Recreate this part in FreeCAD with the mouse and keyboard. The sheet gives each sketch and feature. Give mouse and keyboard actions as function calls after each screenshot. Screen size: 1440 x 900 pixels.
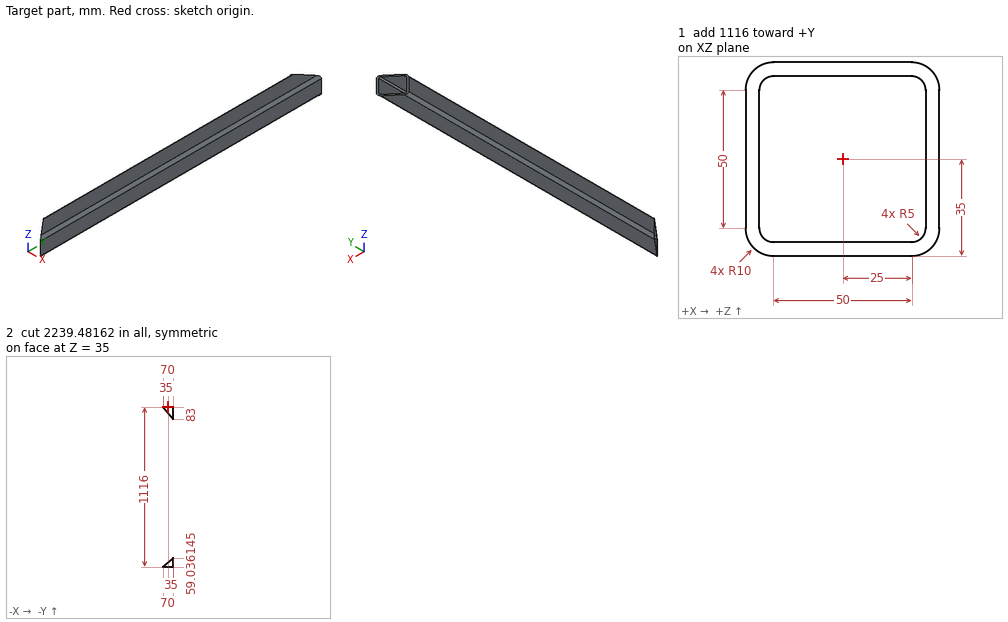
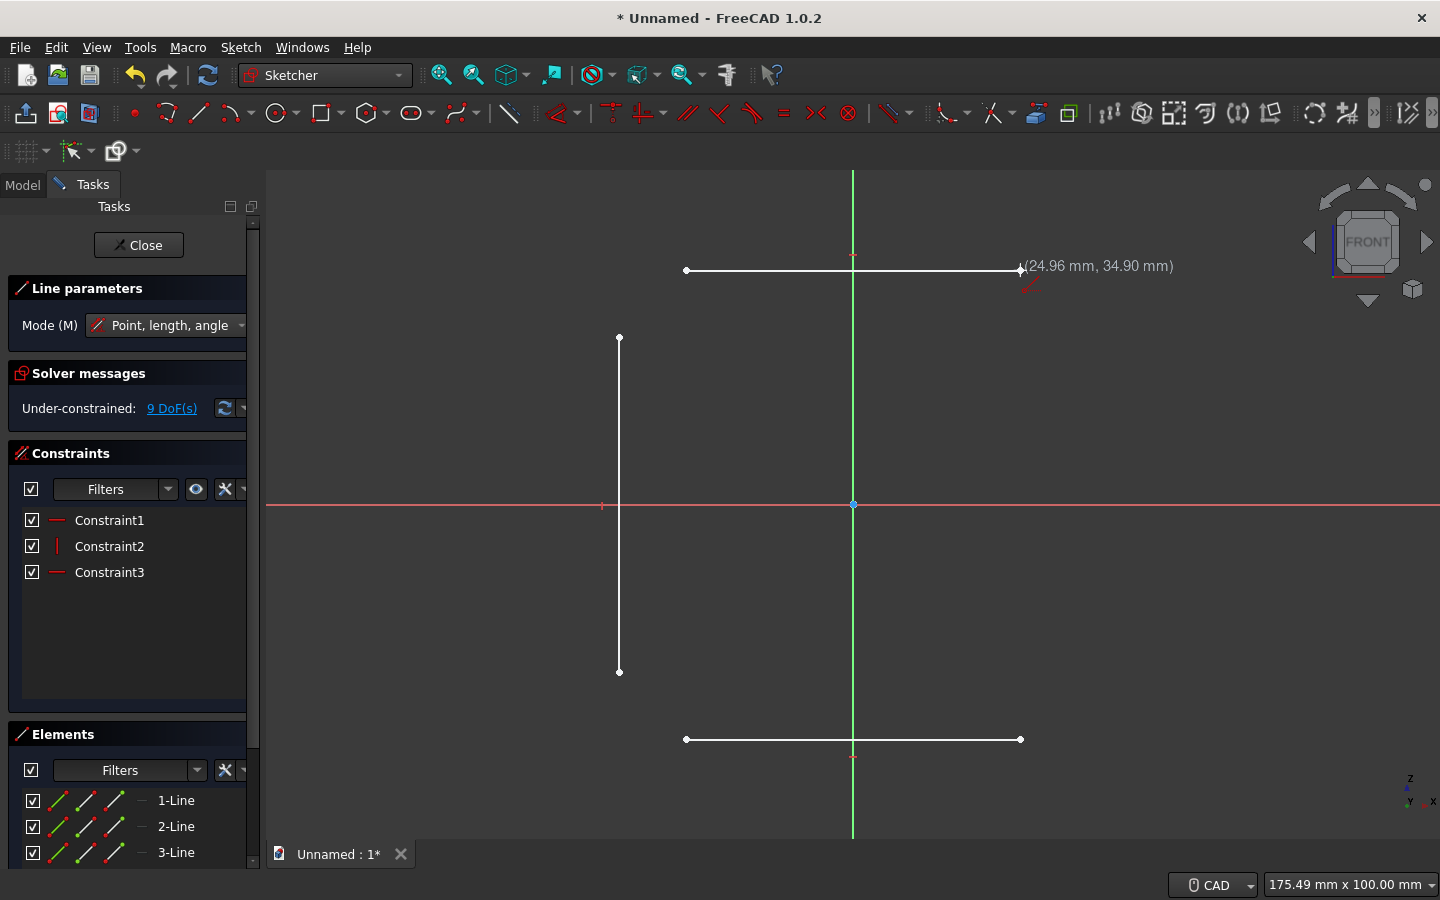
click(1087, 337)
click(1087, 672)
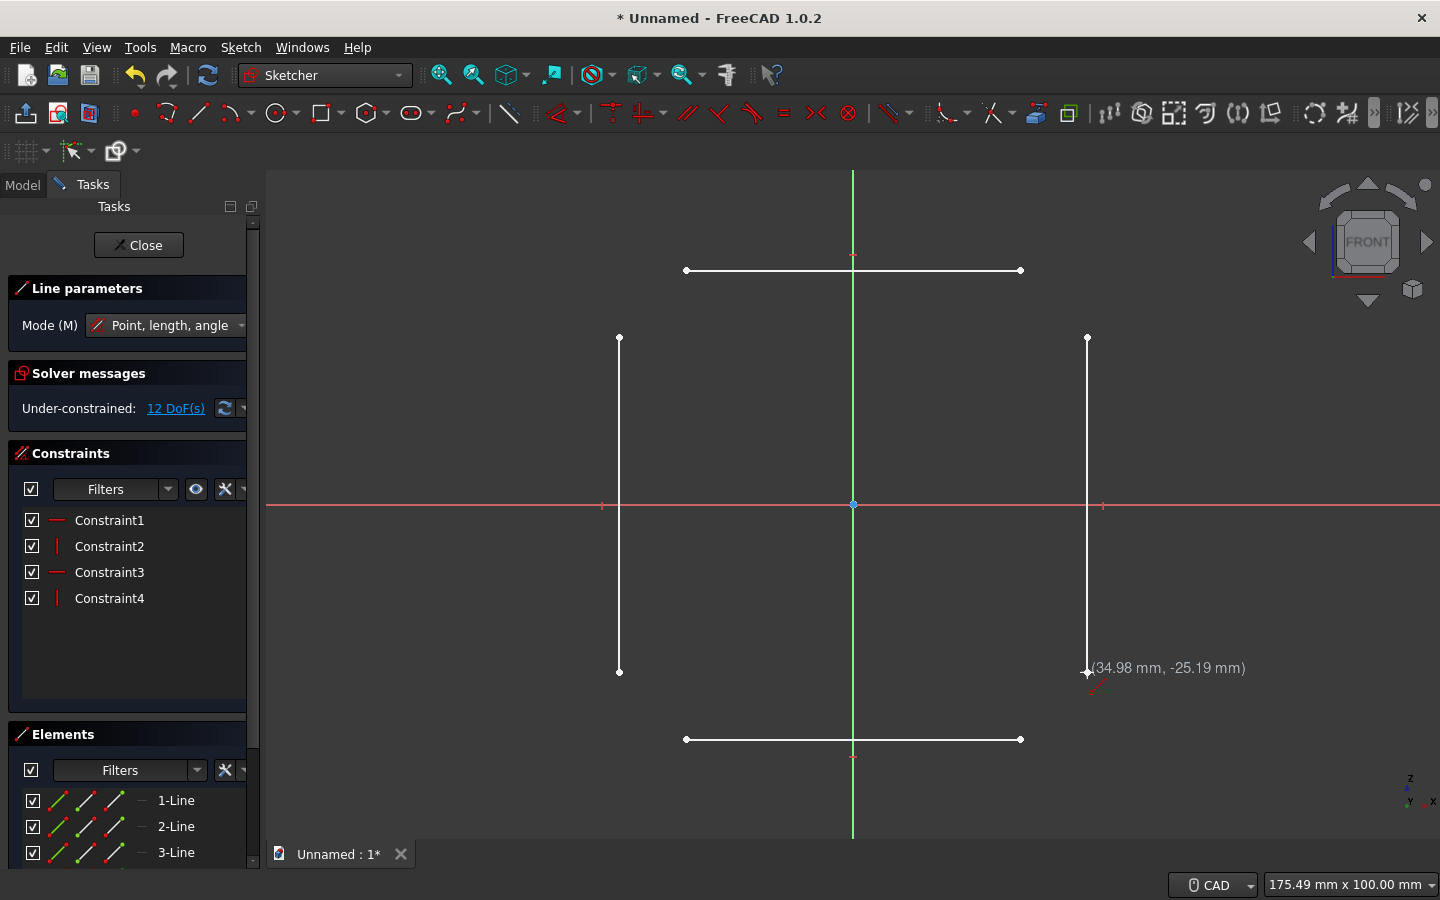
key(g)
key(3)
key(a)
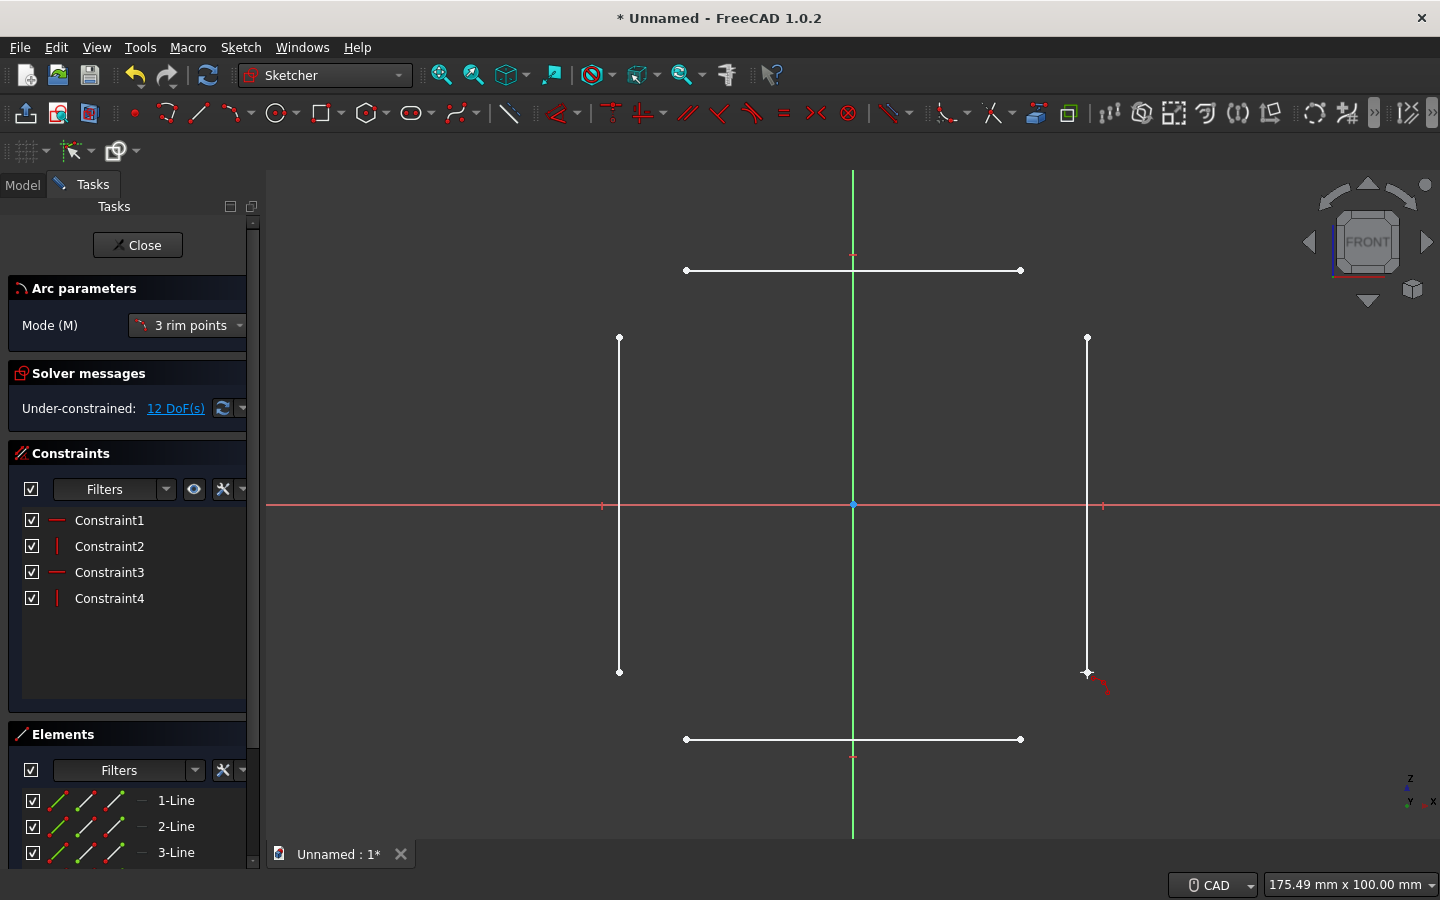
click(686, 740)
click(619, 673)
click(638, 719)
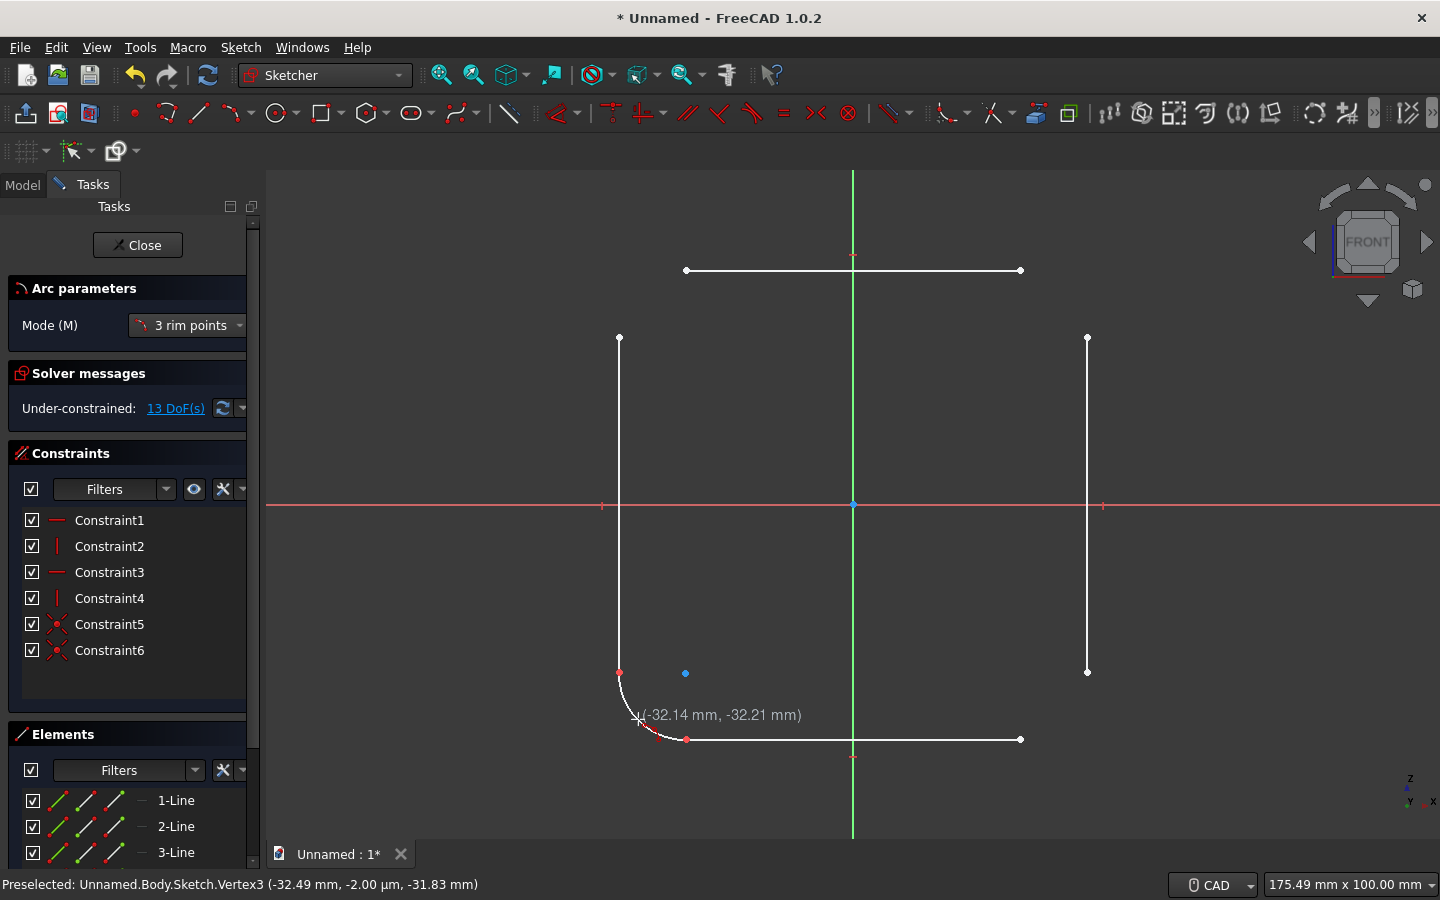
click(619, 338)
click(686, 271)
click(638, 290)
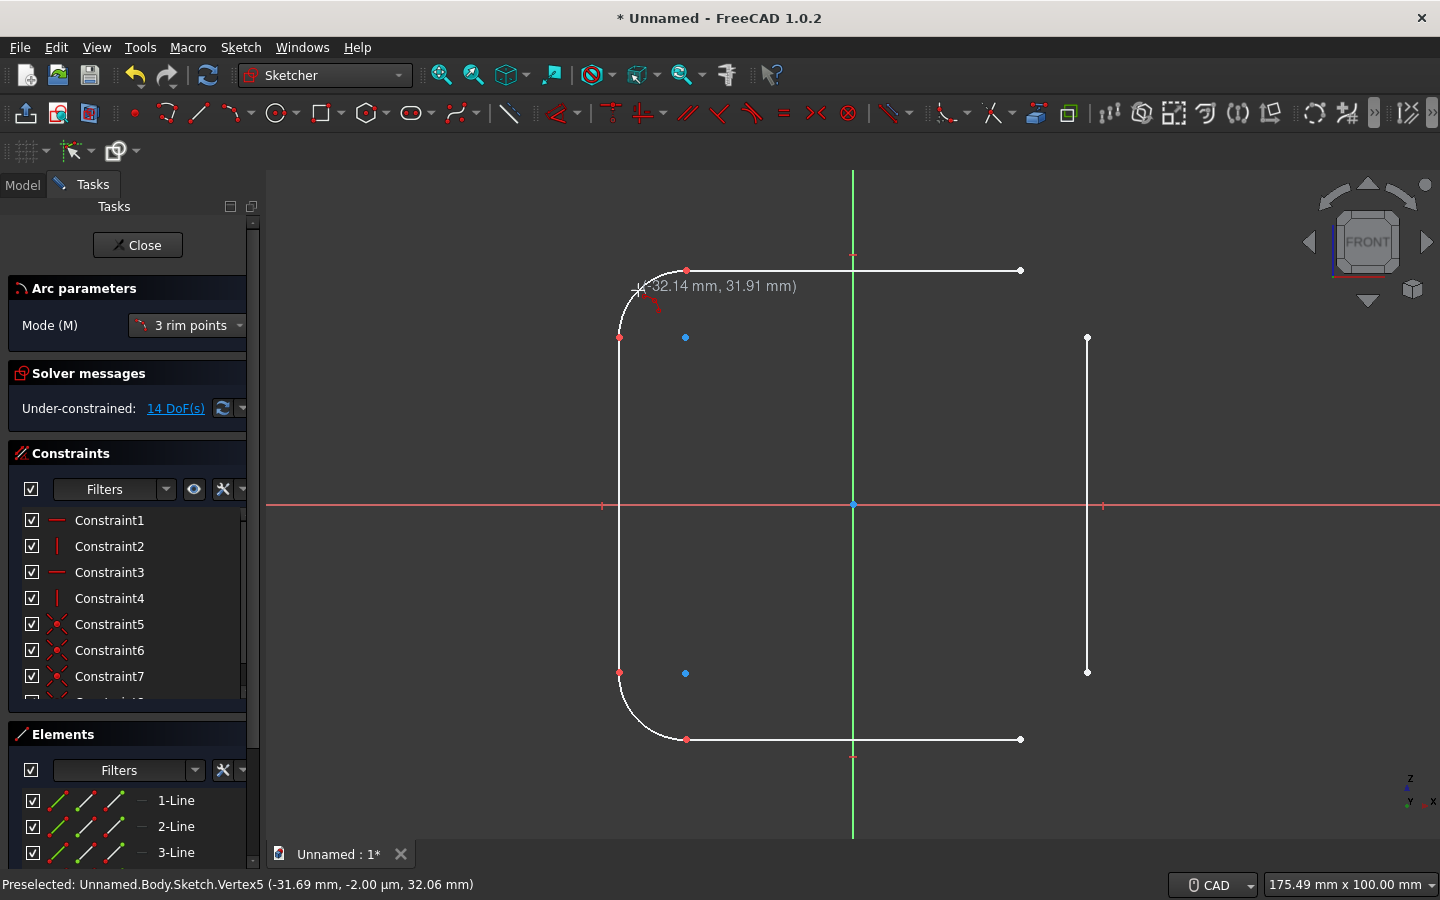
click(1020, 271)
click(1087, 338)
click(1068, 290)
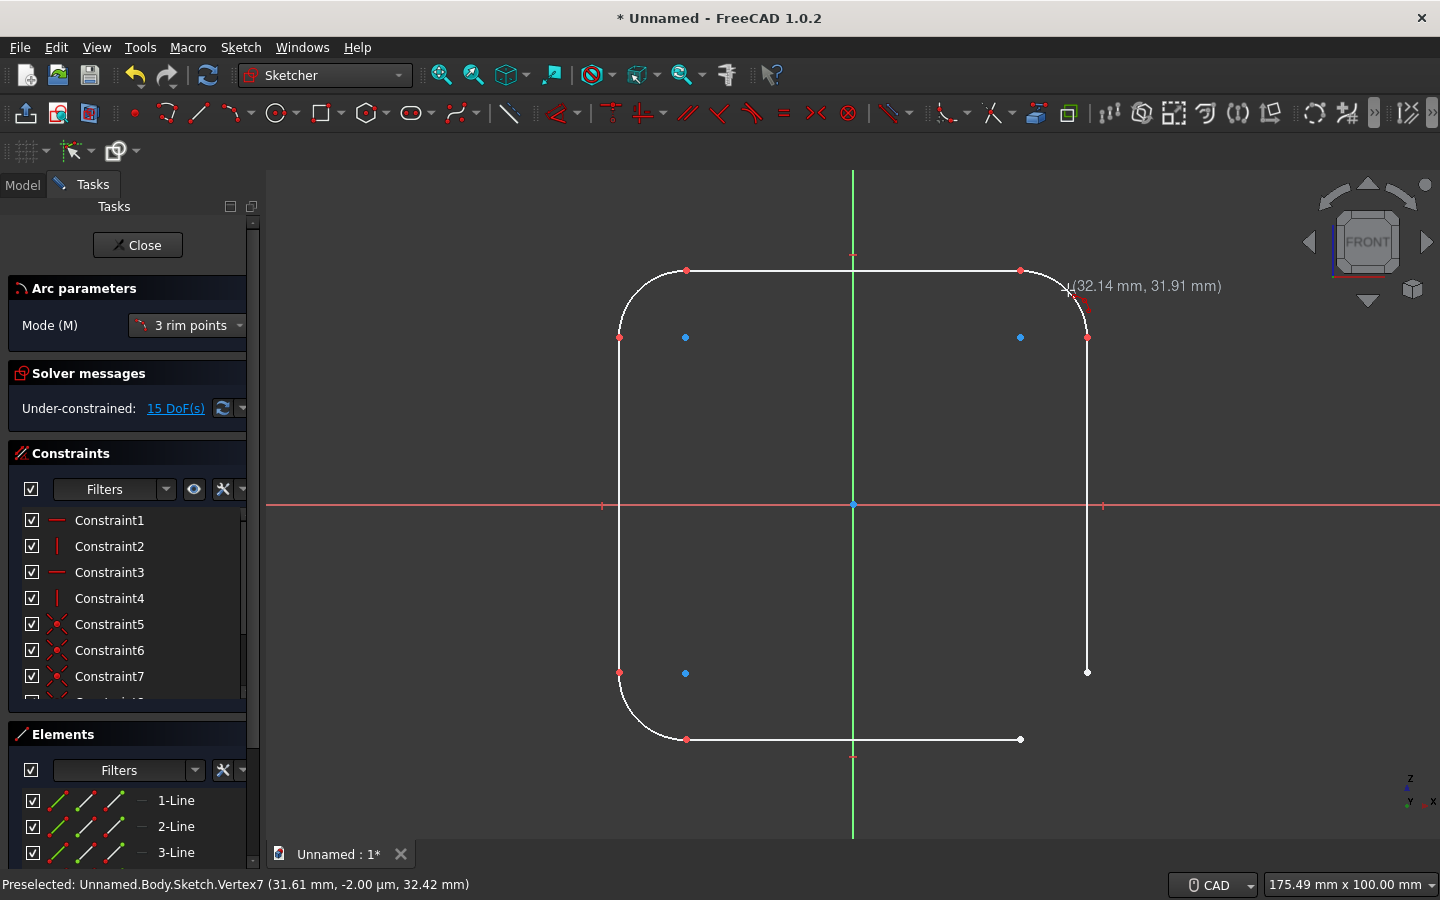
click(1087, 673)
click(1020, 740)
click(1068, 719)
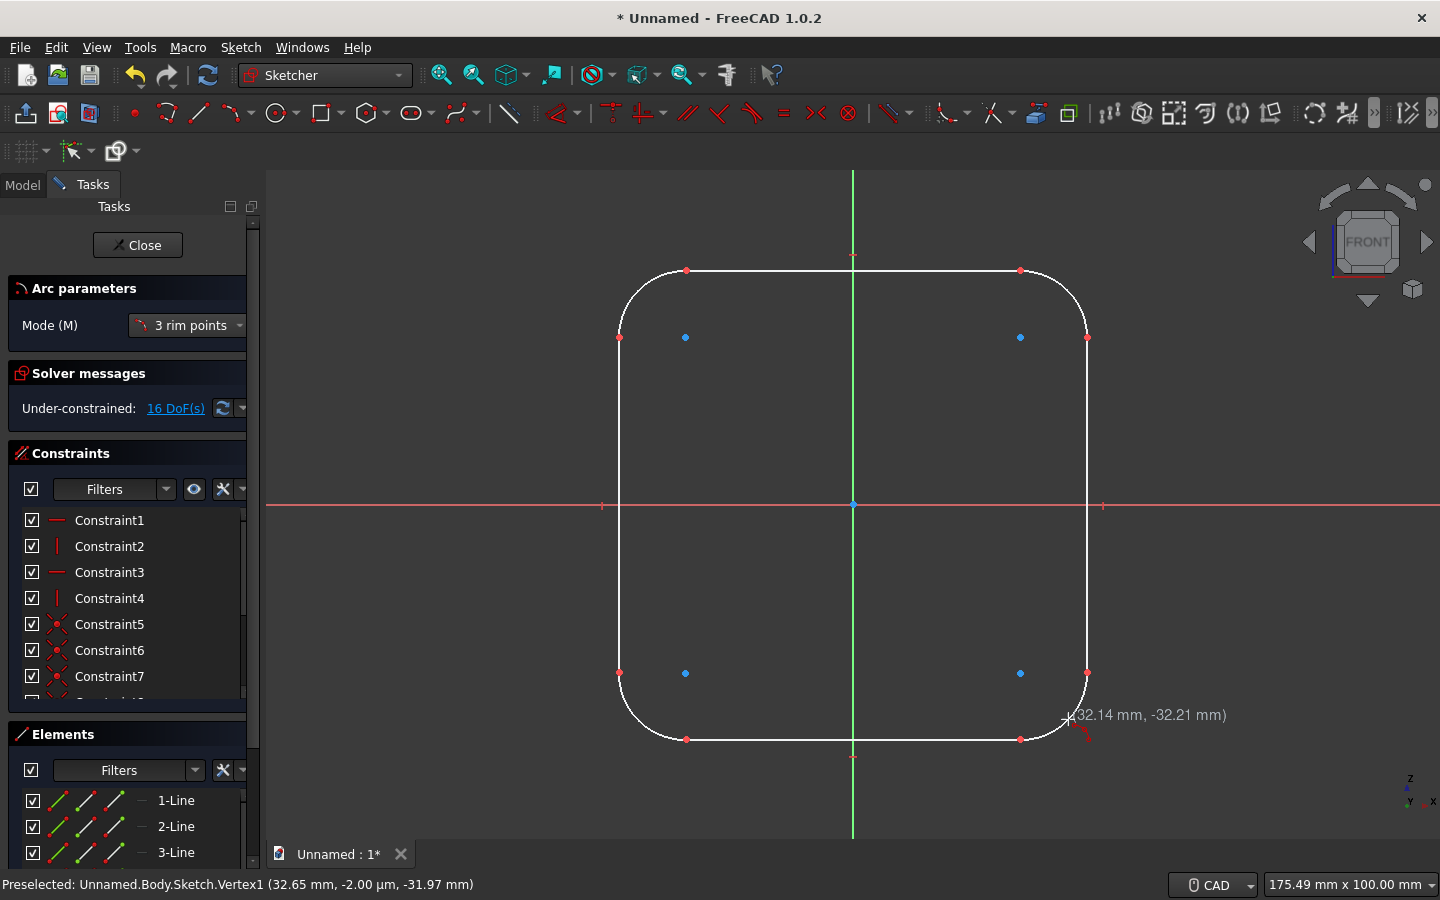
key(g)
key(l)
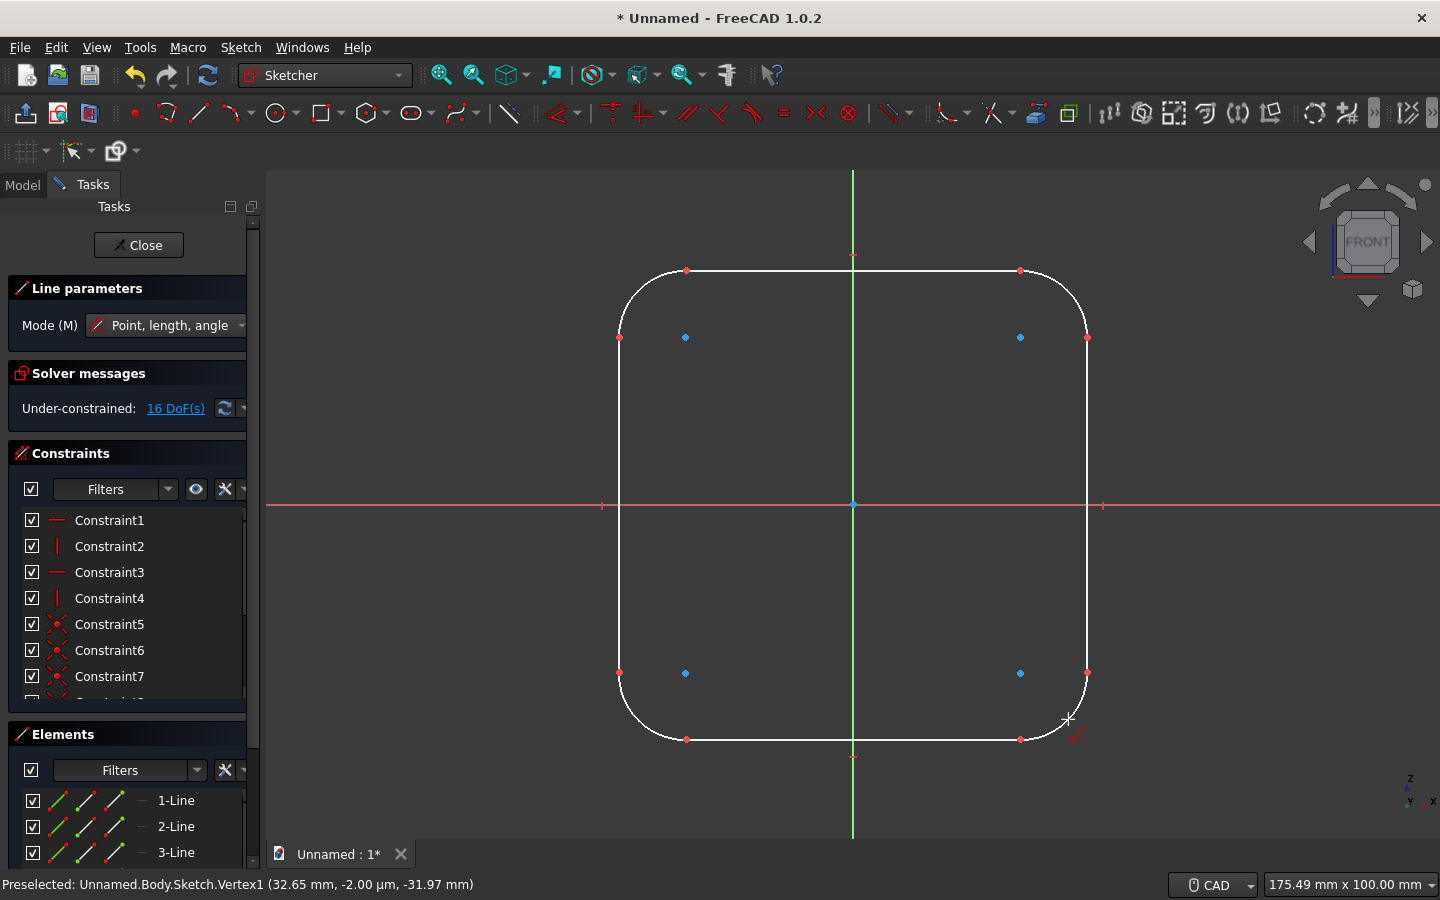
click(686, 705)
click(1020, 705)